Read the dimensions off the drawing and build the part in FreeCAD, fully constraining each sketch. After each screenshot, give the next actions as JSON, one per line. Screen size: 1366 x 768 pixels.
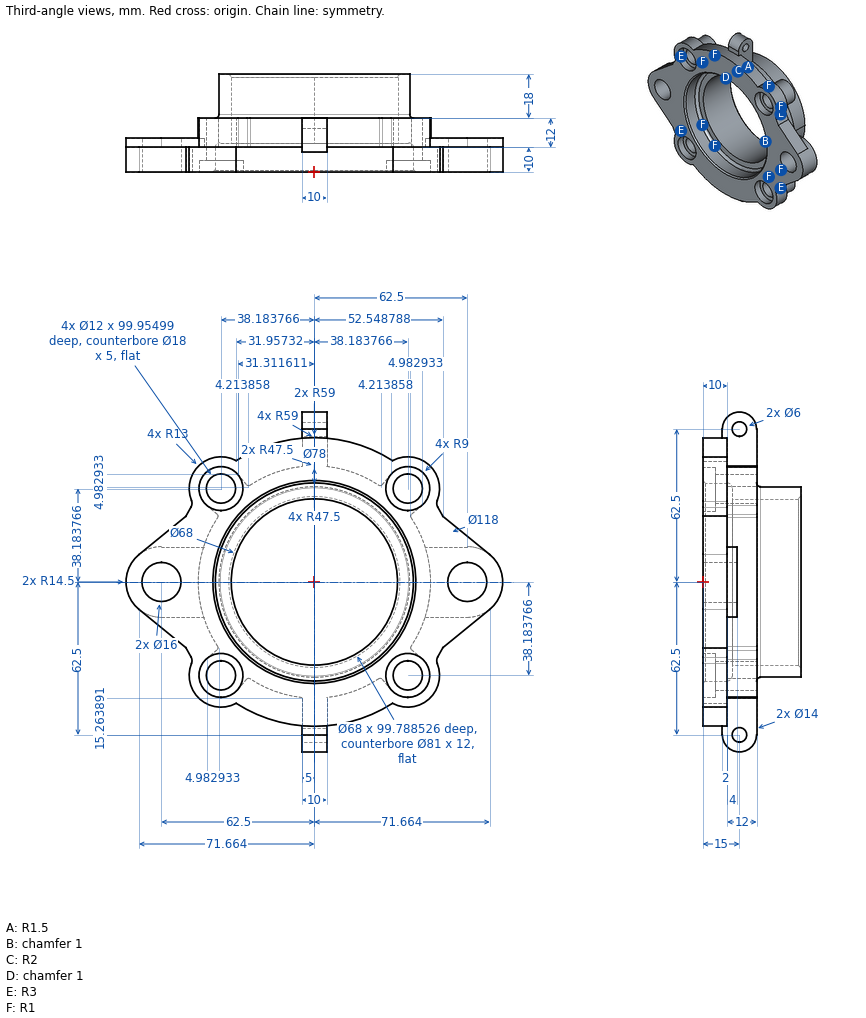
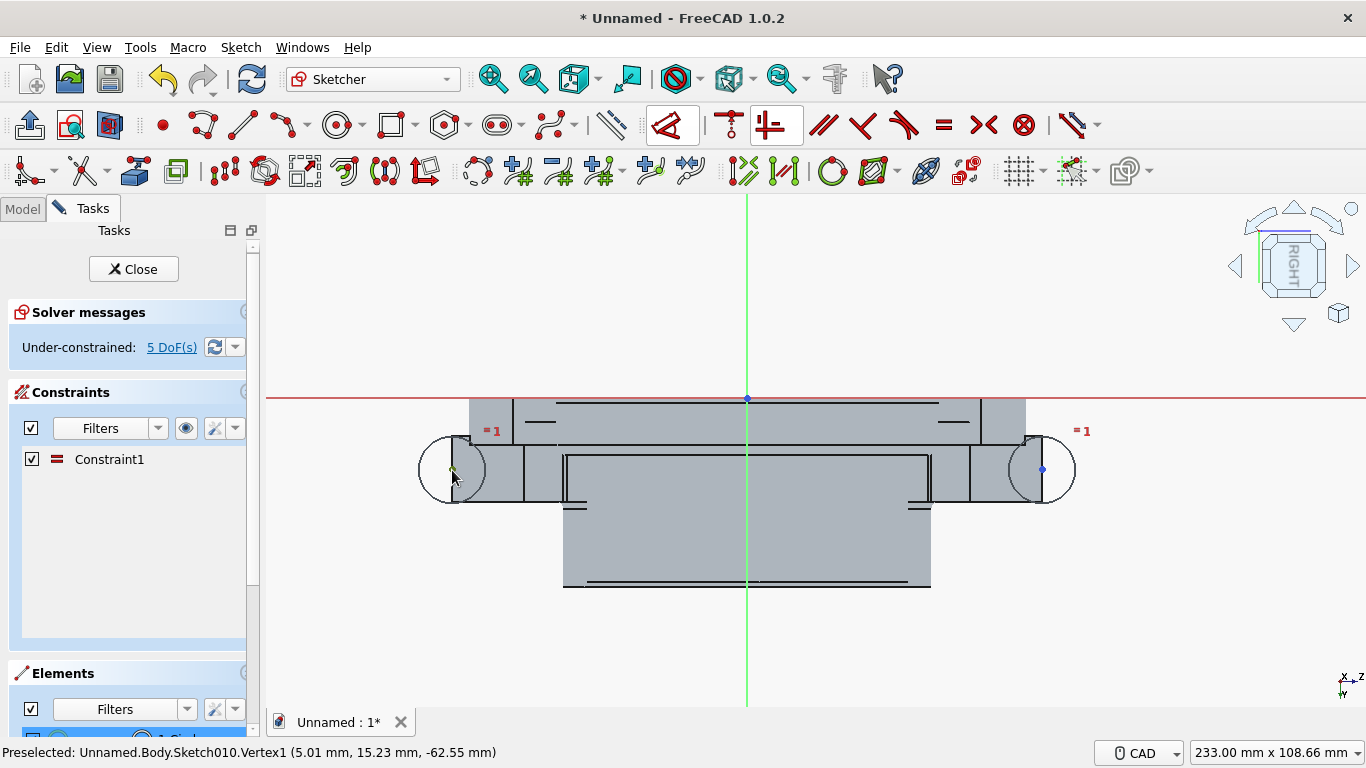
{"action": "left_click", "coordinate": [1042, 470]}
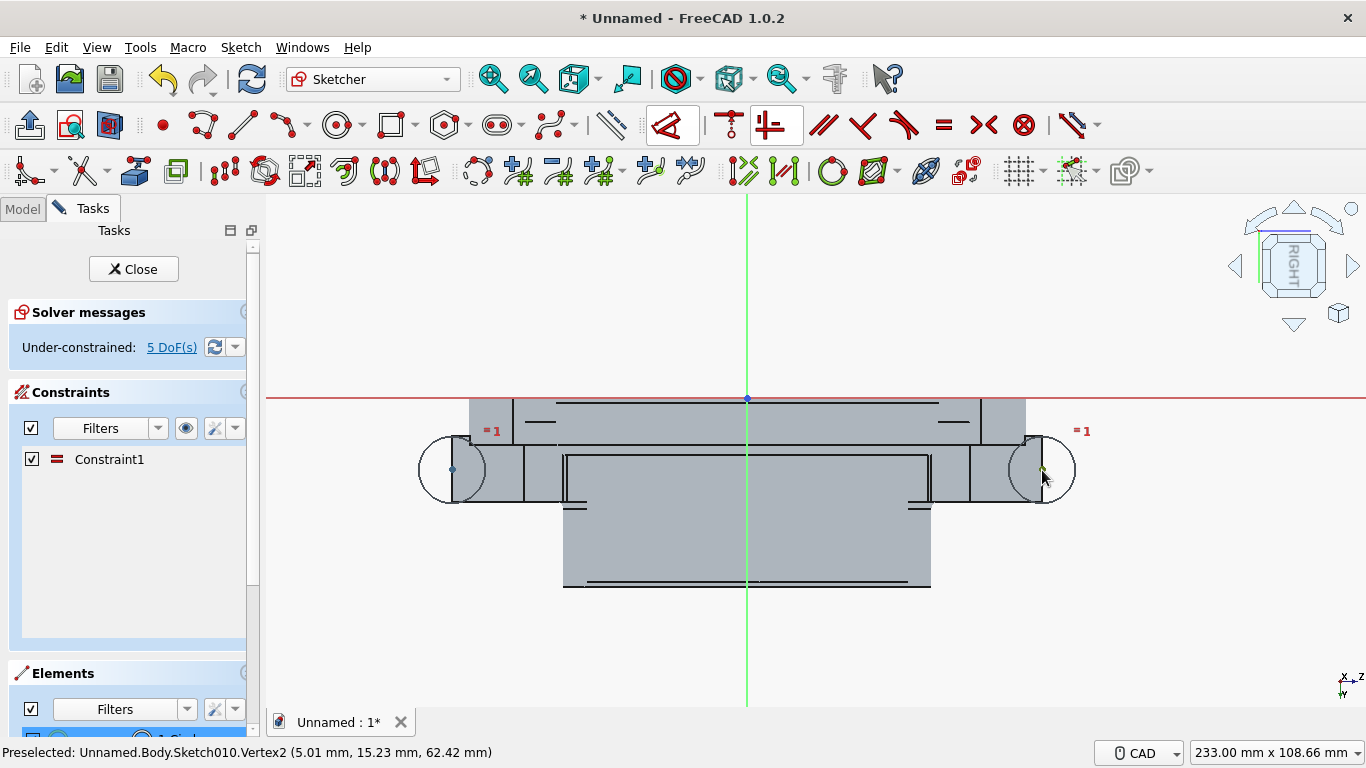
{"action": "left_click", "coordinate": [798, 126]}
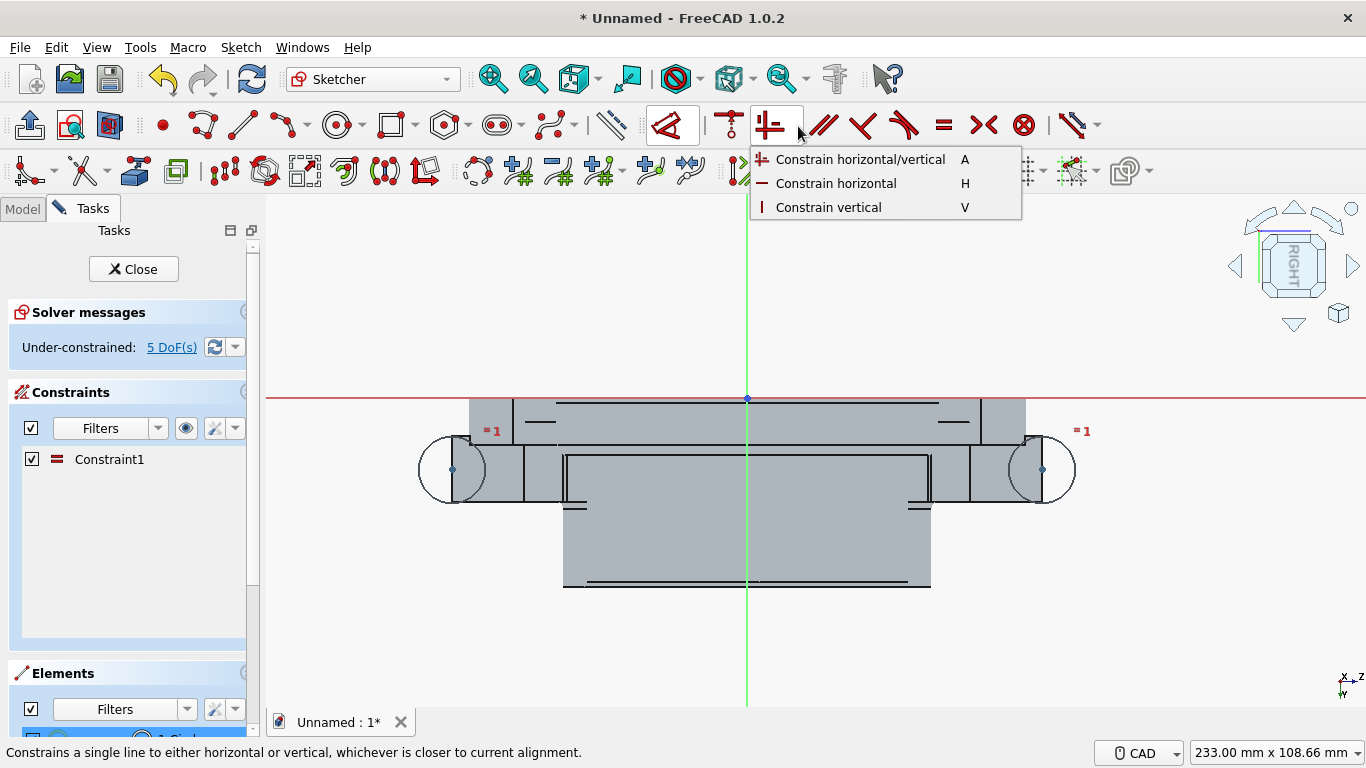
{"action": "left_click", "coordinate": [886, 183]}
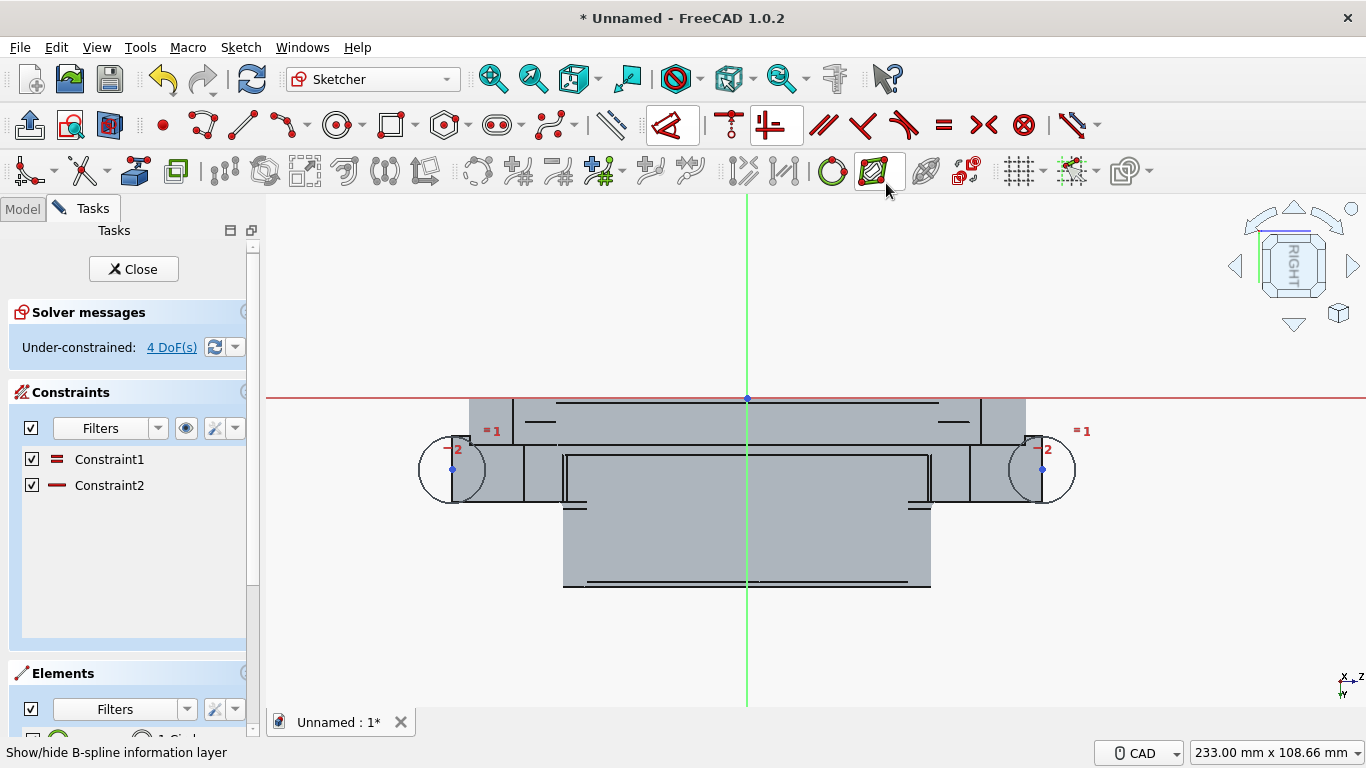
{"action": "left_click", "coordinate": [475, 446]}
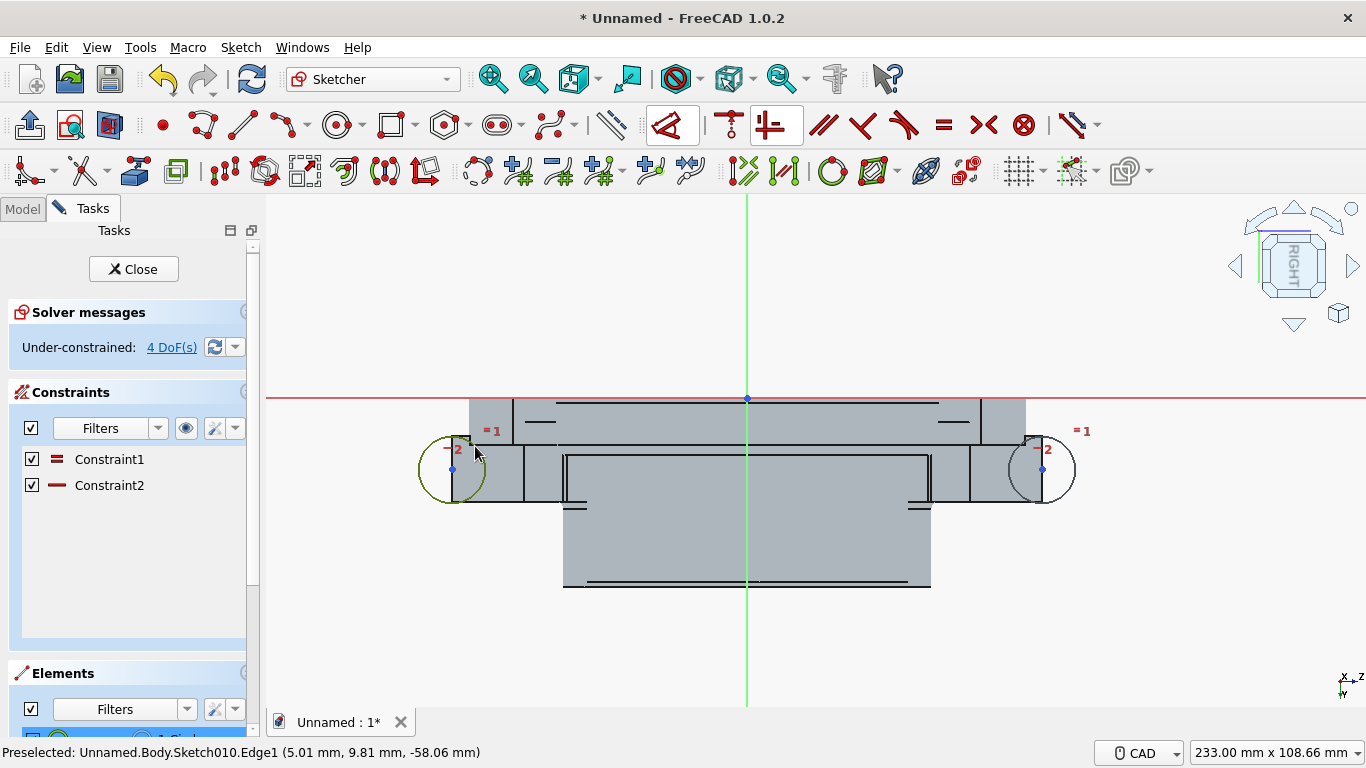
{"action": "left_click", "coordinate": [694, 126]}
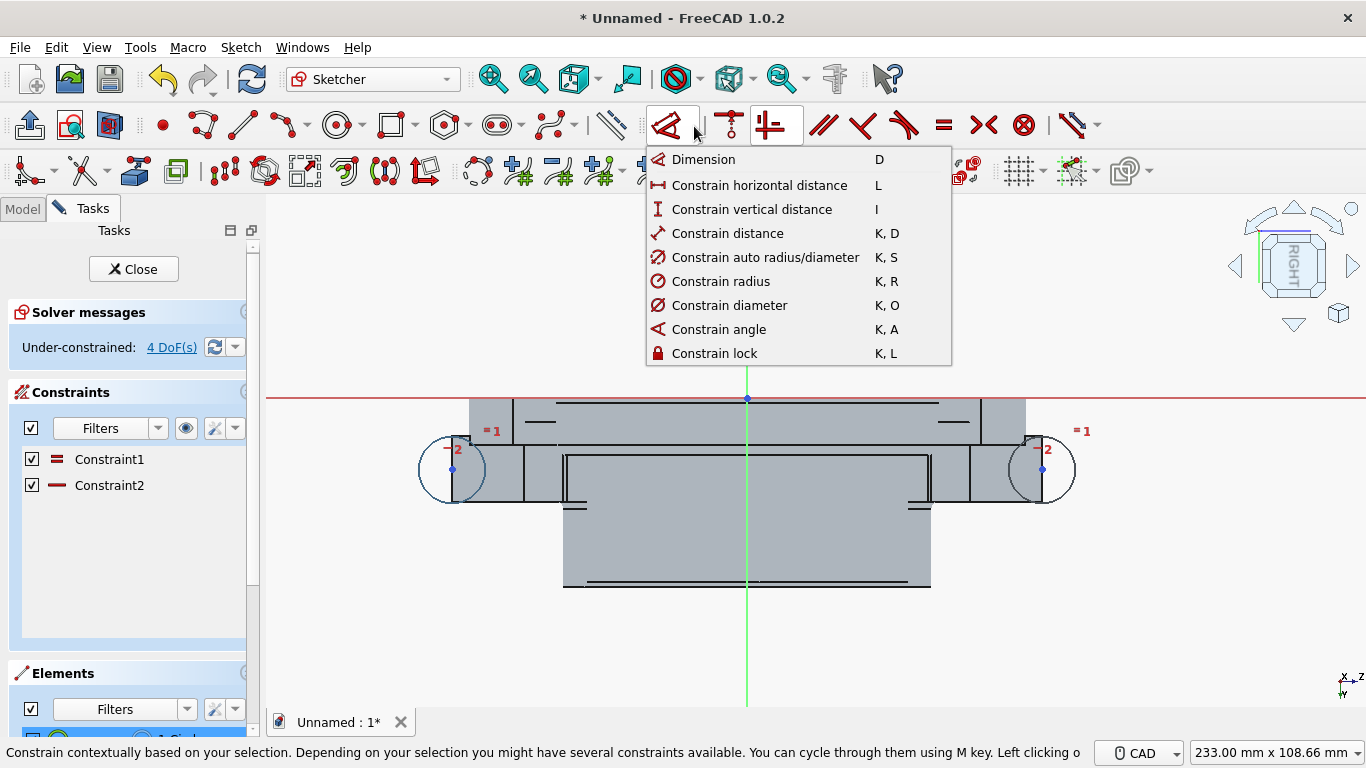
{"action": "left_click", "coordinate": [799, 305]}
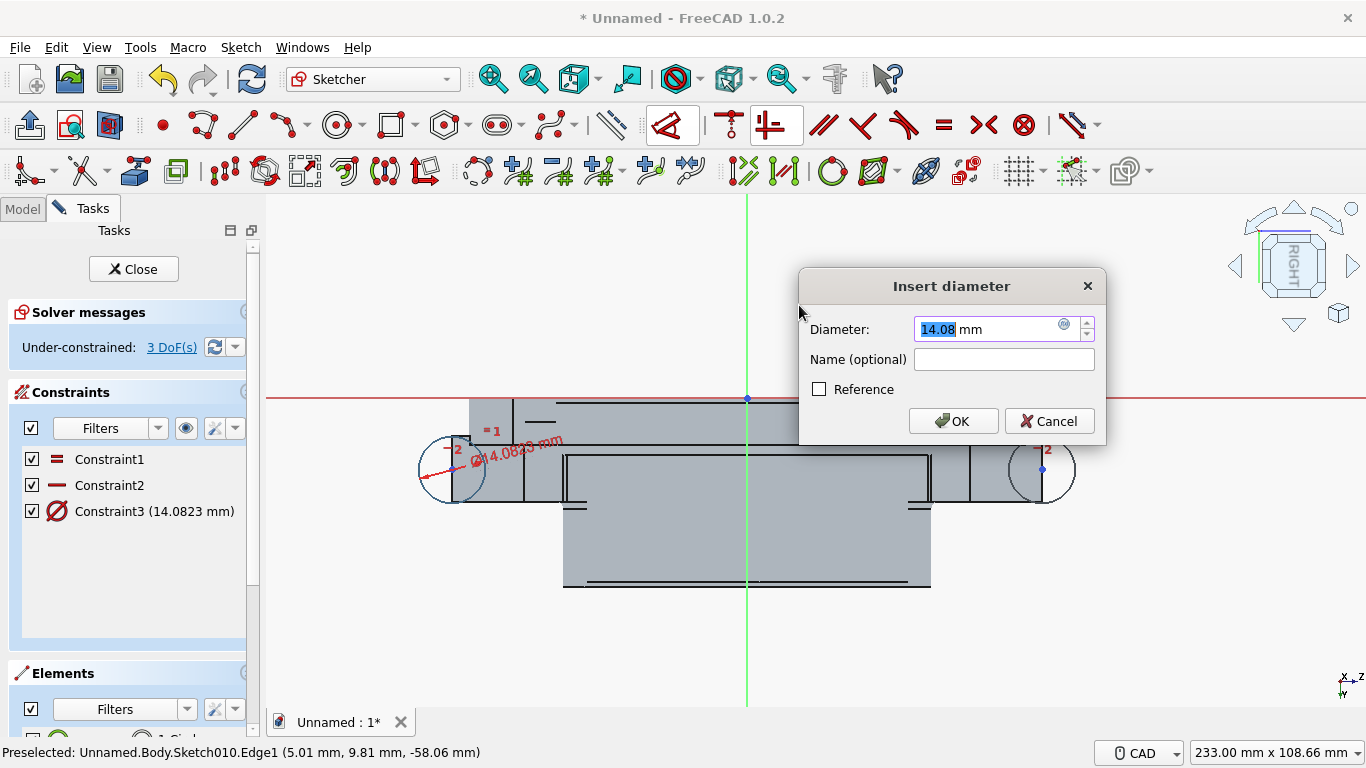
{"action": "type", "text": "14"}
{"action": "key", "text": "Return"}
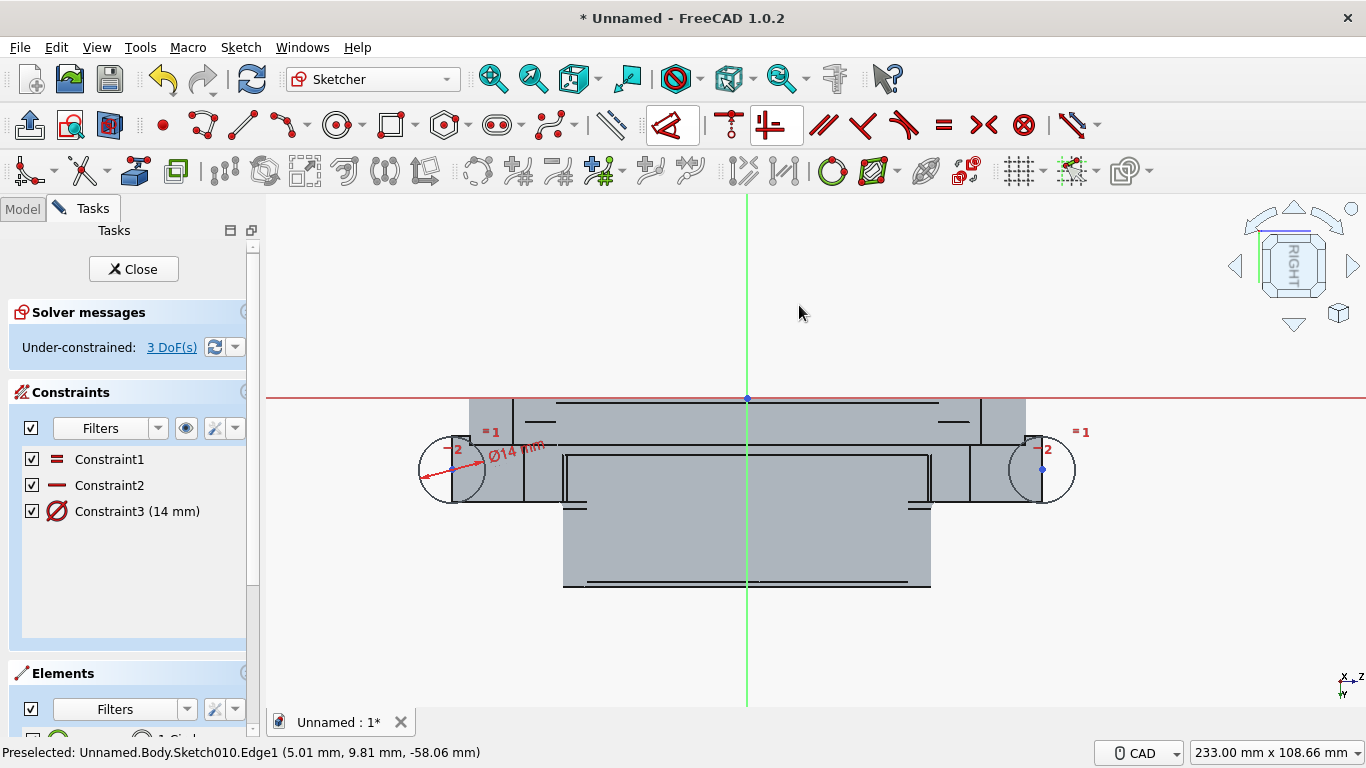
{"action": "left_click", "coordinate": [452, 470]}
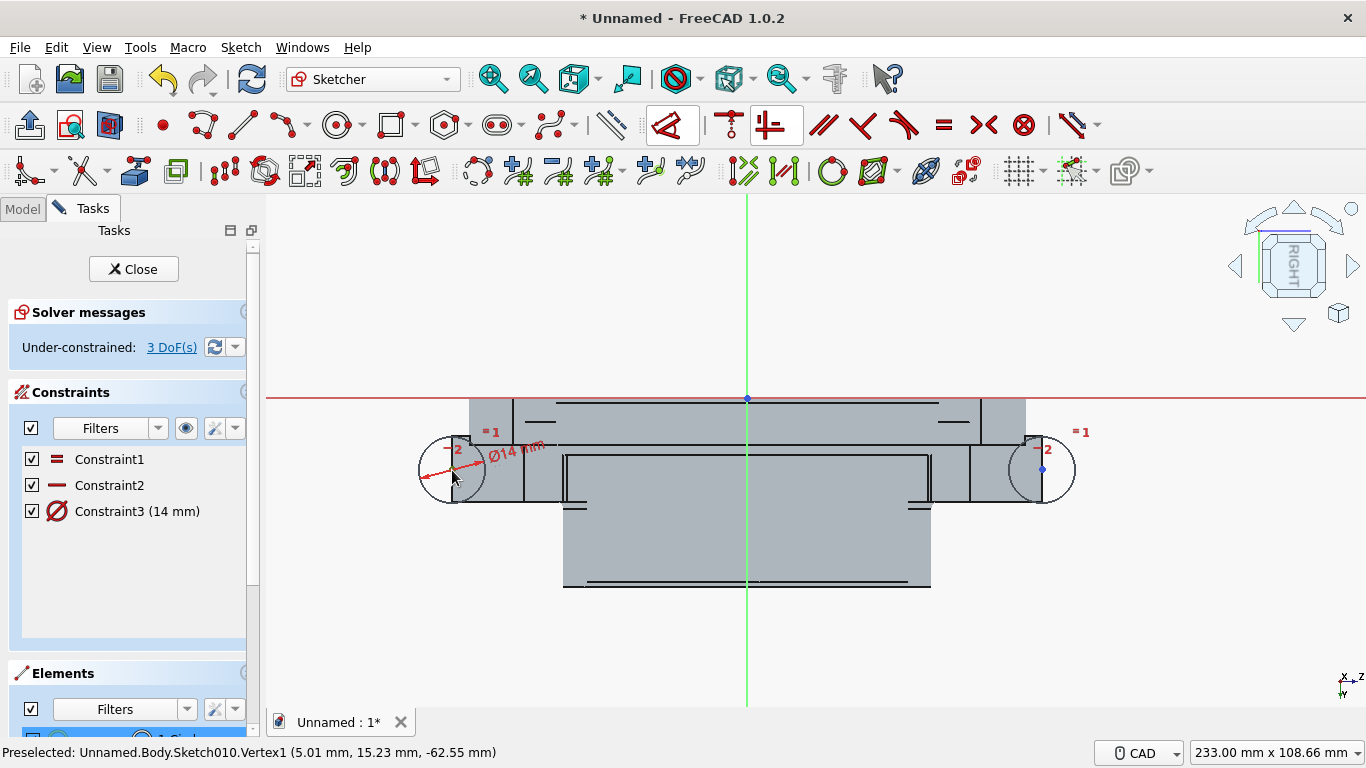
{"action": "left_click", "coordinate": [694, 126]}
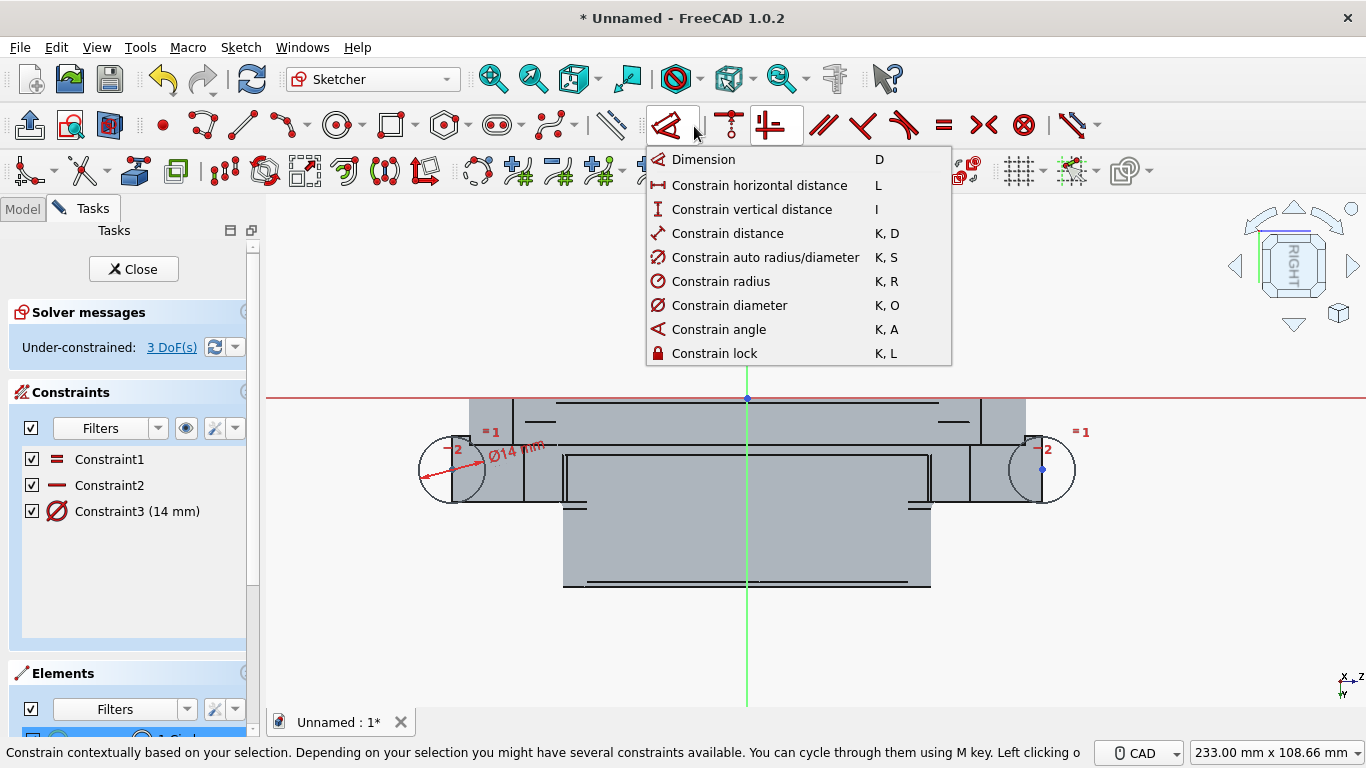
{"action": "left_click", "coordinate": [799, 209]}